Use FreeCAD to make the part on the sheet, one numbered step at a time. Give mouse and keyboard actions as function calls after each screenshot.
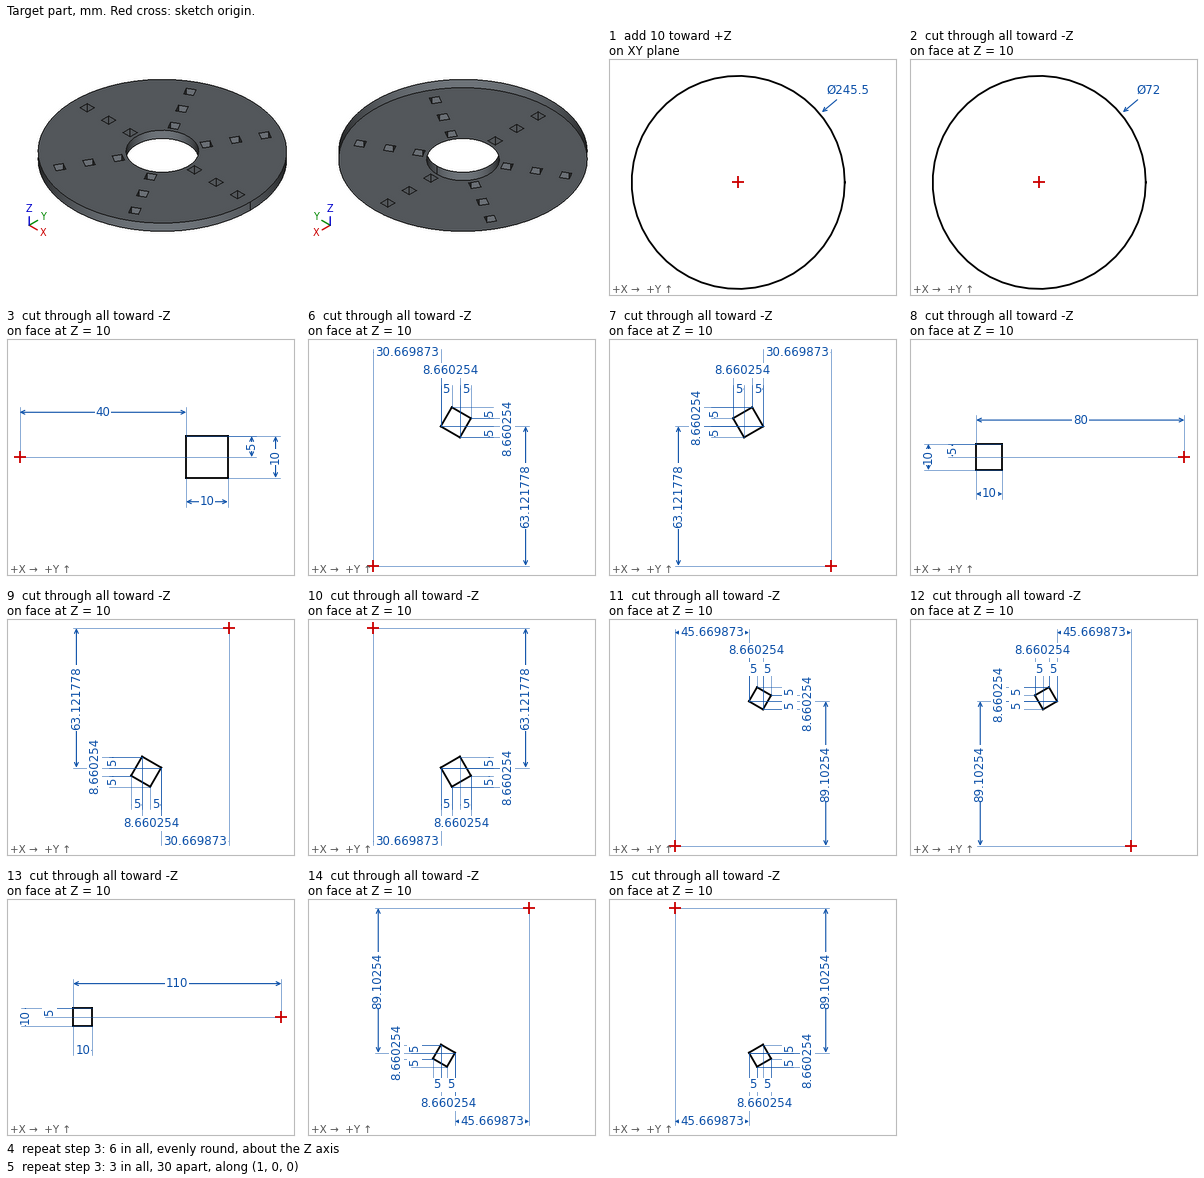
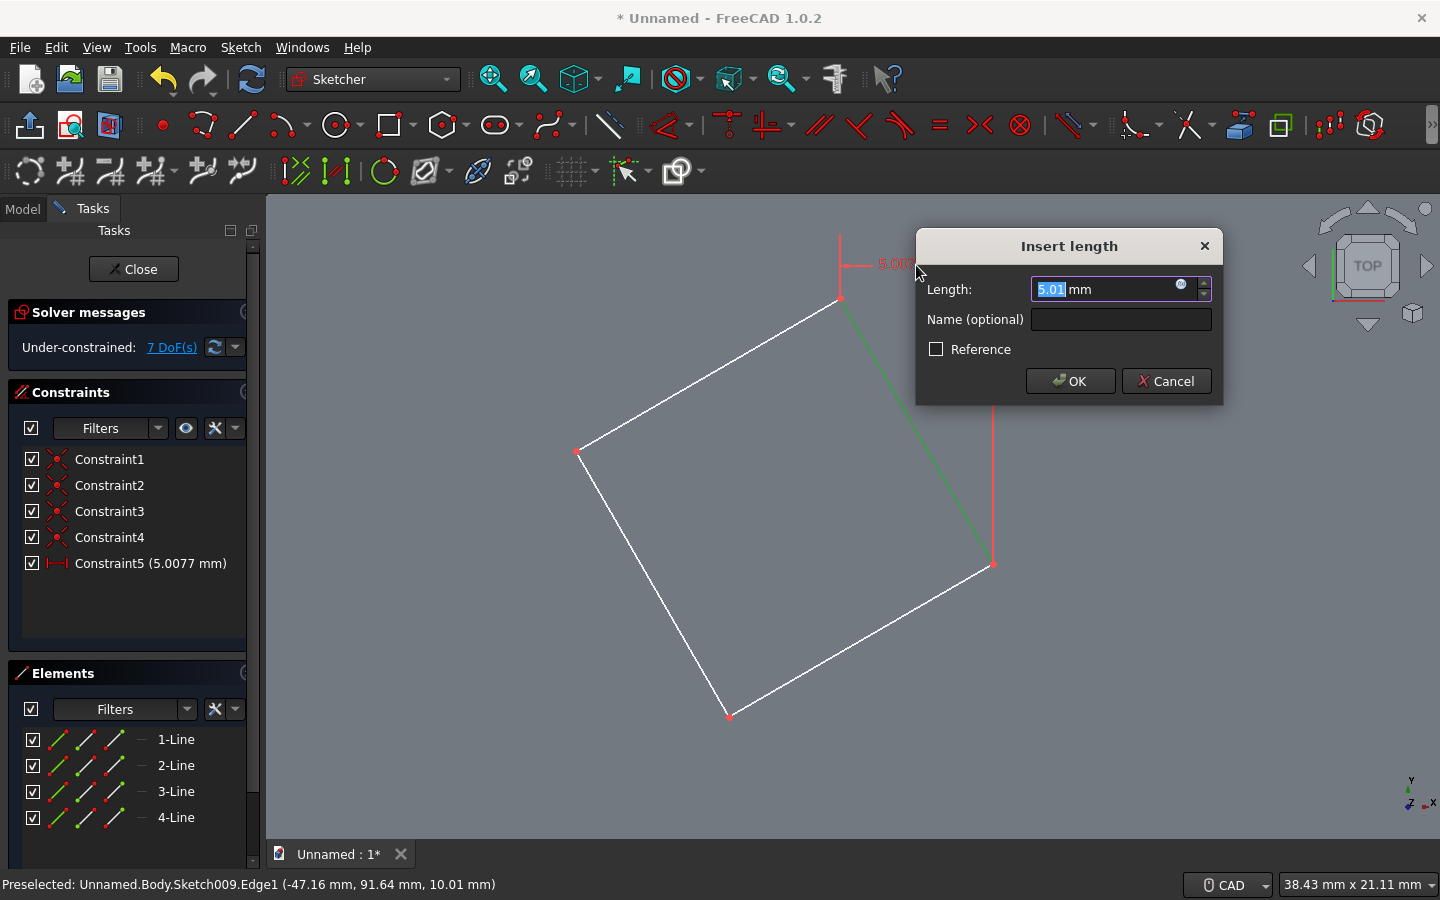
text(5)
key(Return)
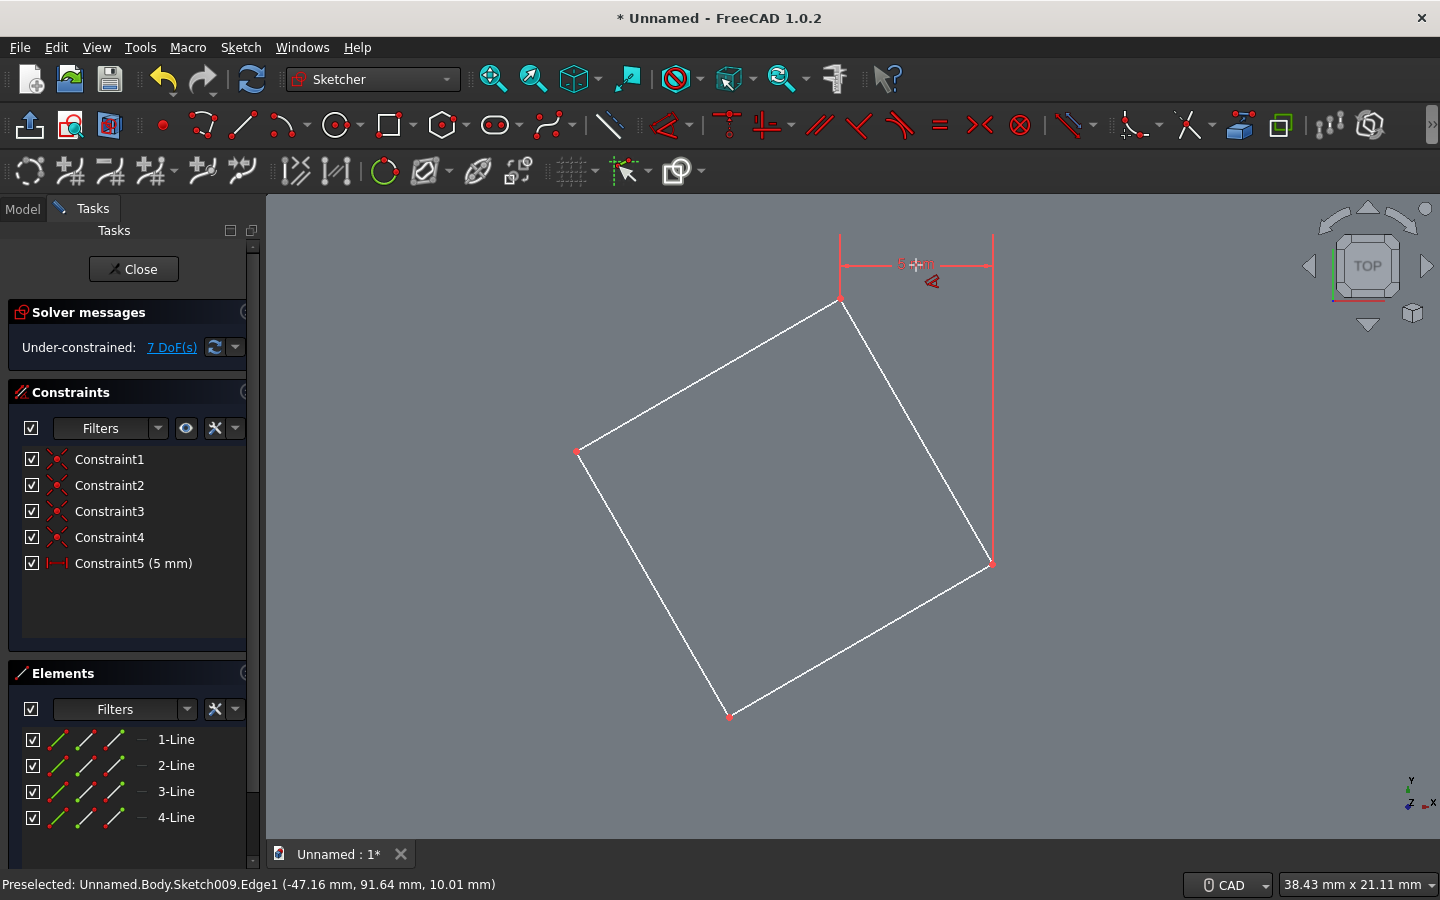
click(761, 345)
click(542, 375)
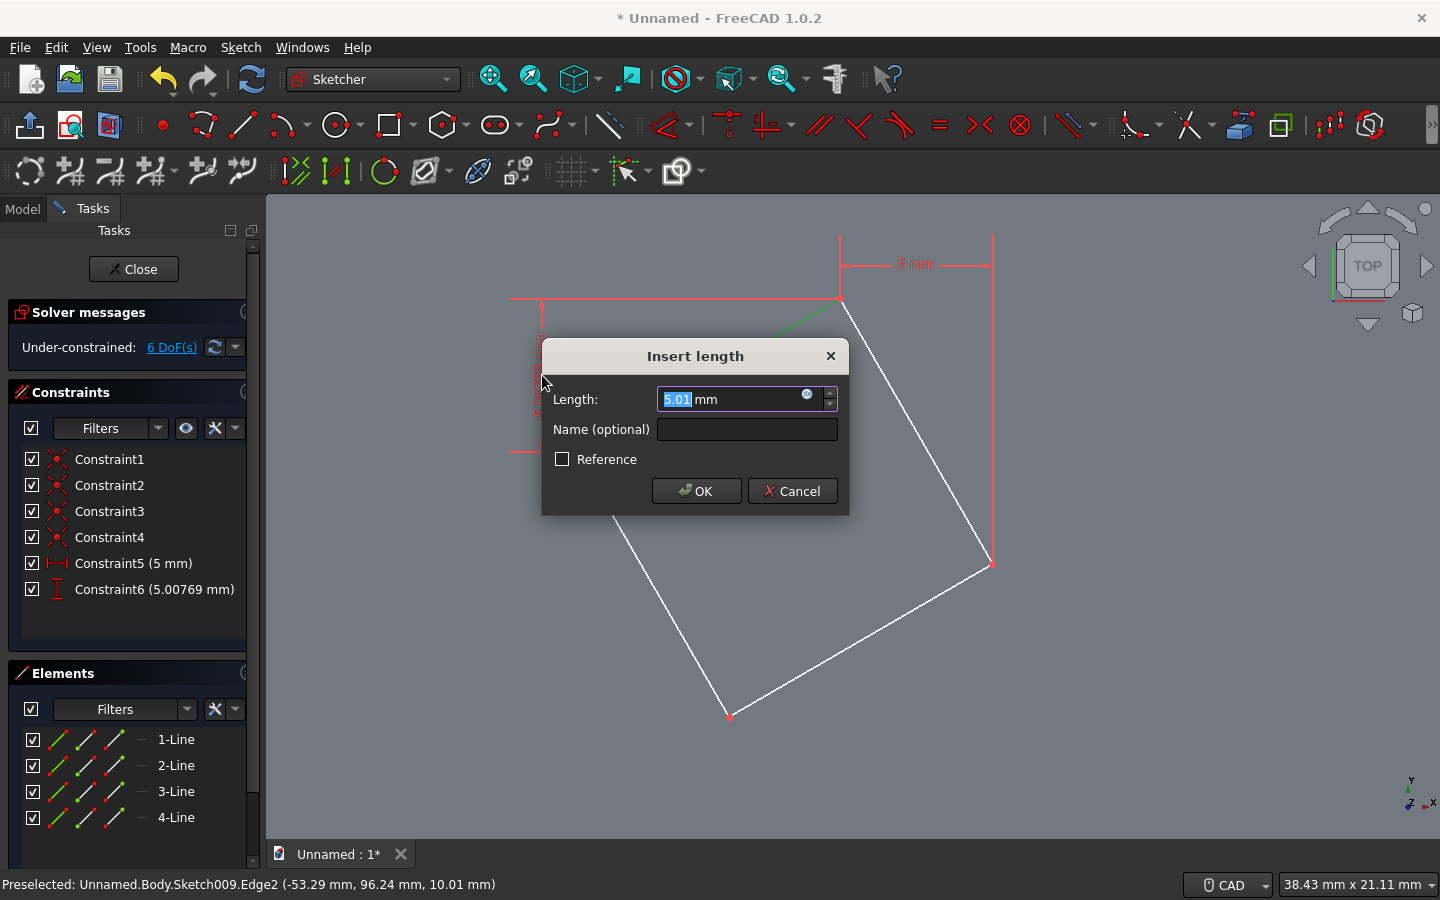
text(5)
key(Return)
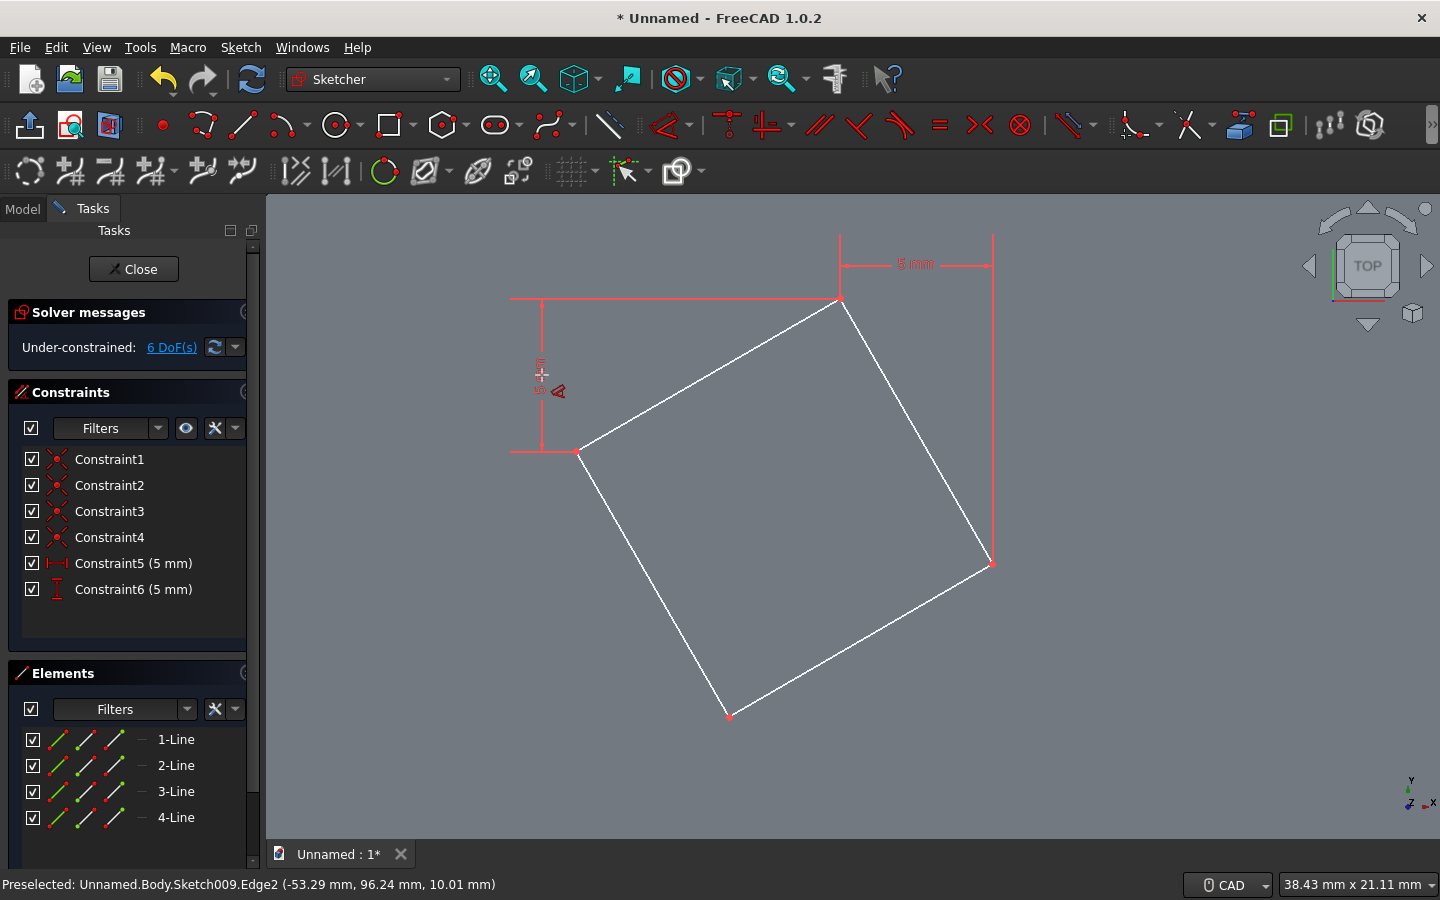
click(622, 531)
click(653, 751)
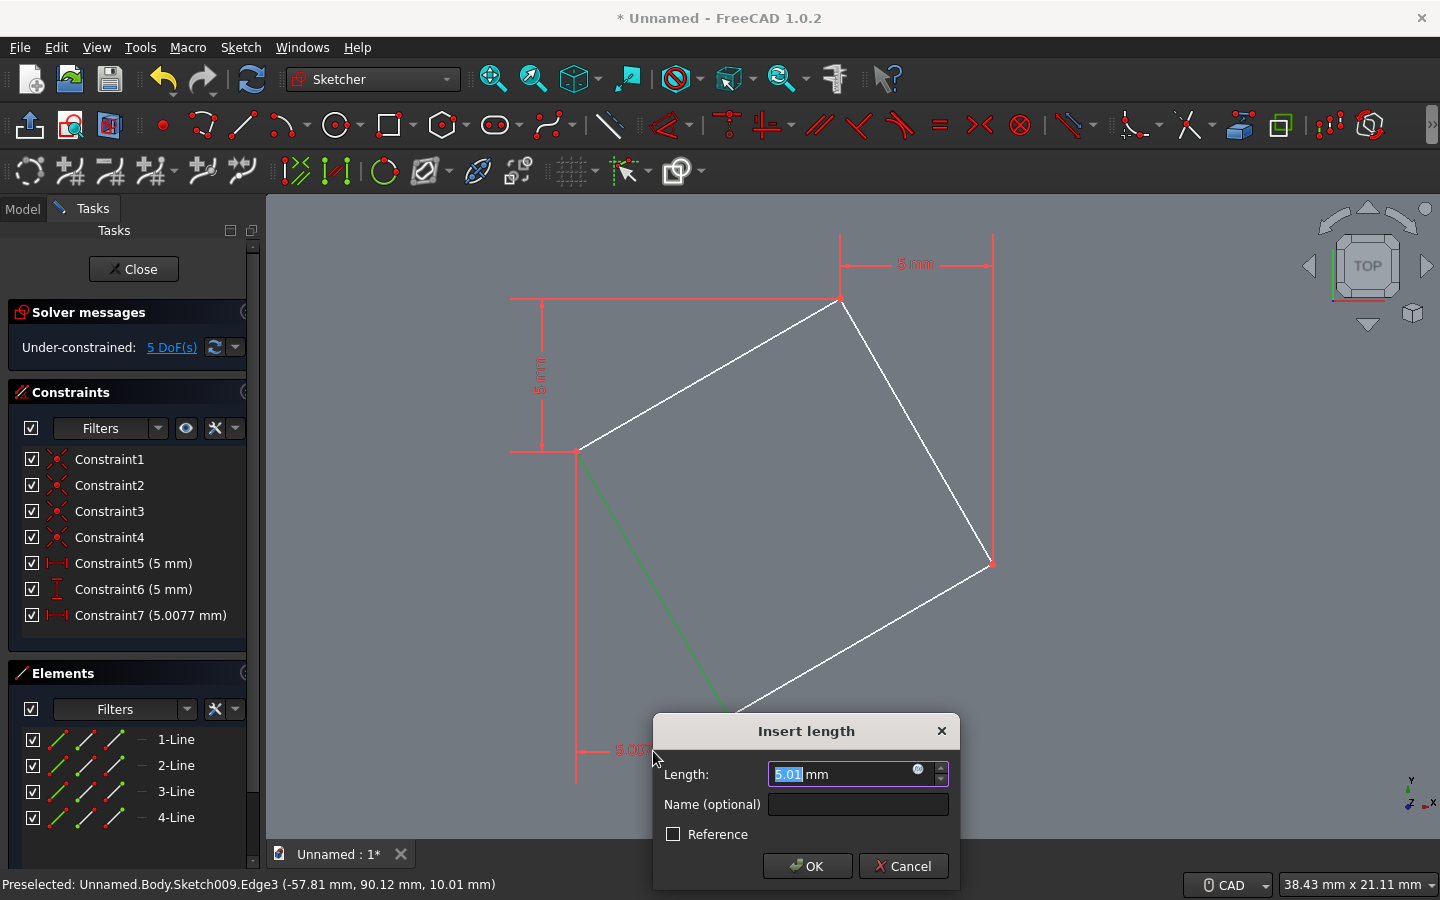
text(5)
key(Return)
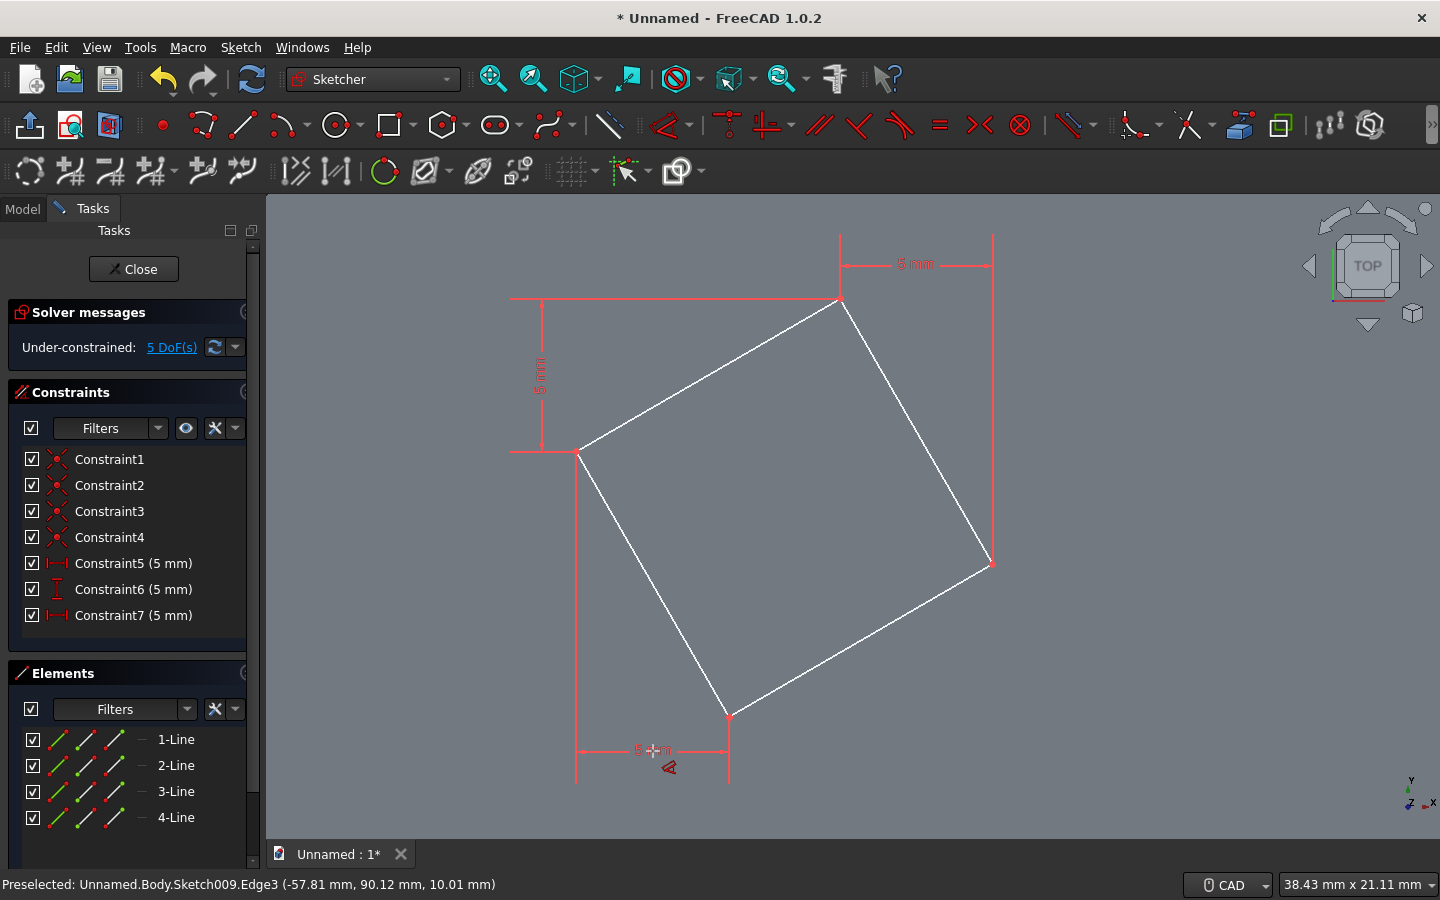
click(808, 671)
click(1027, 641)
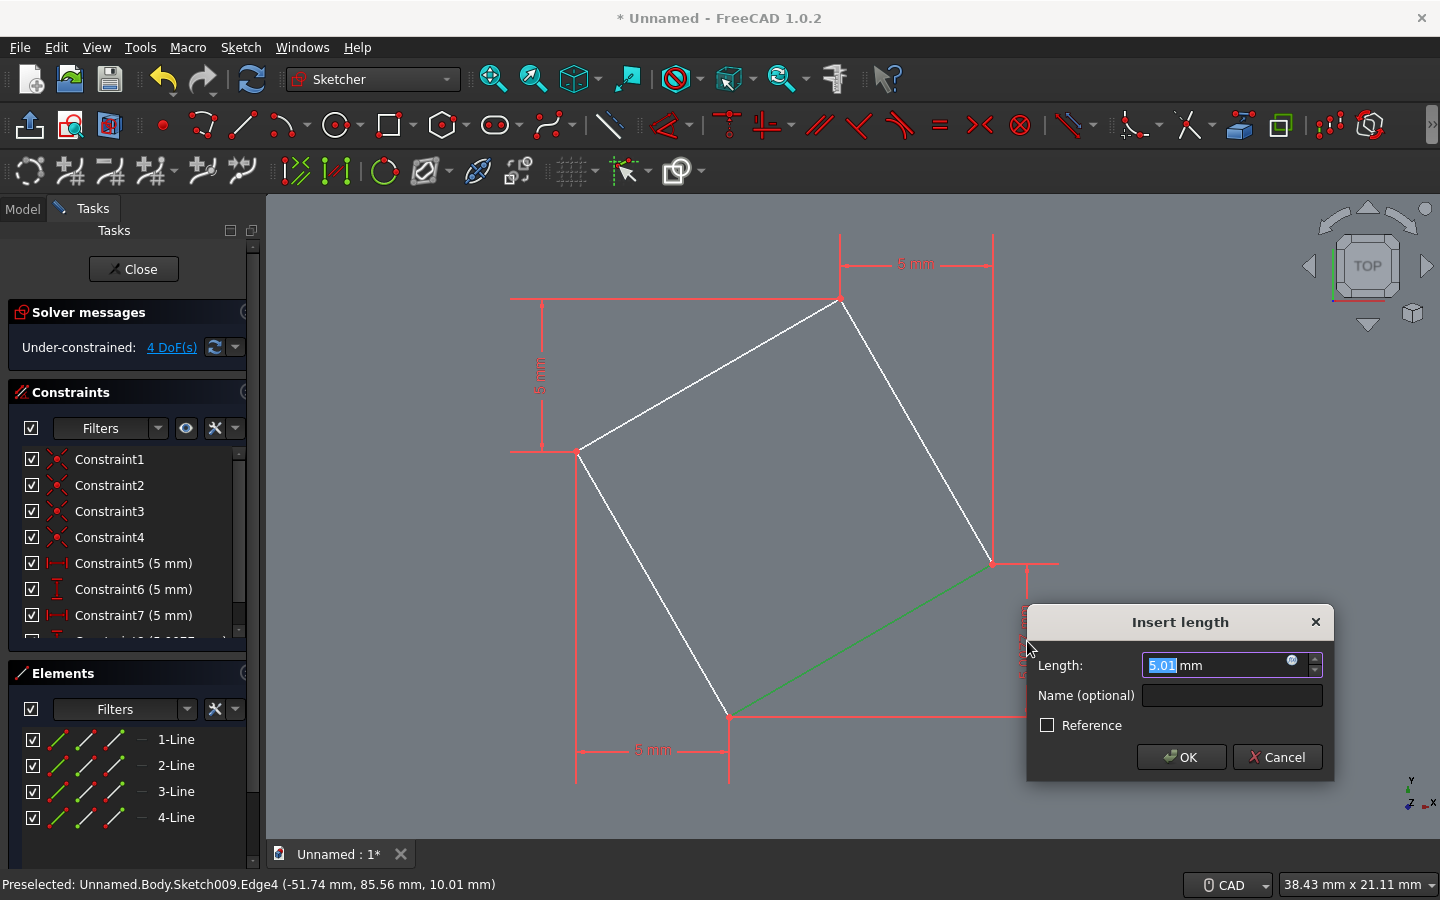
text(5)
key(Return)